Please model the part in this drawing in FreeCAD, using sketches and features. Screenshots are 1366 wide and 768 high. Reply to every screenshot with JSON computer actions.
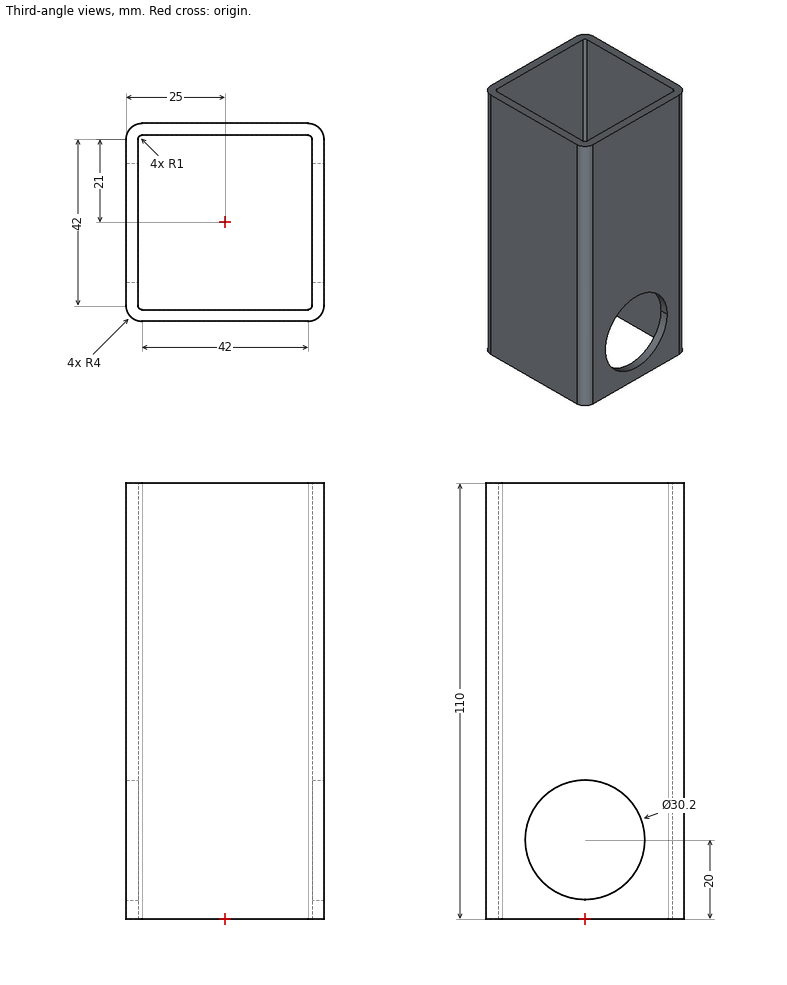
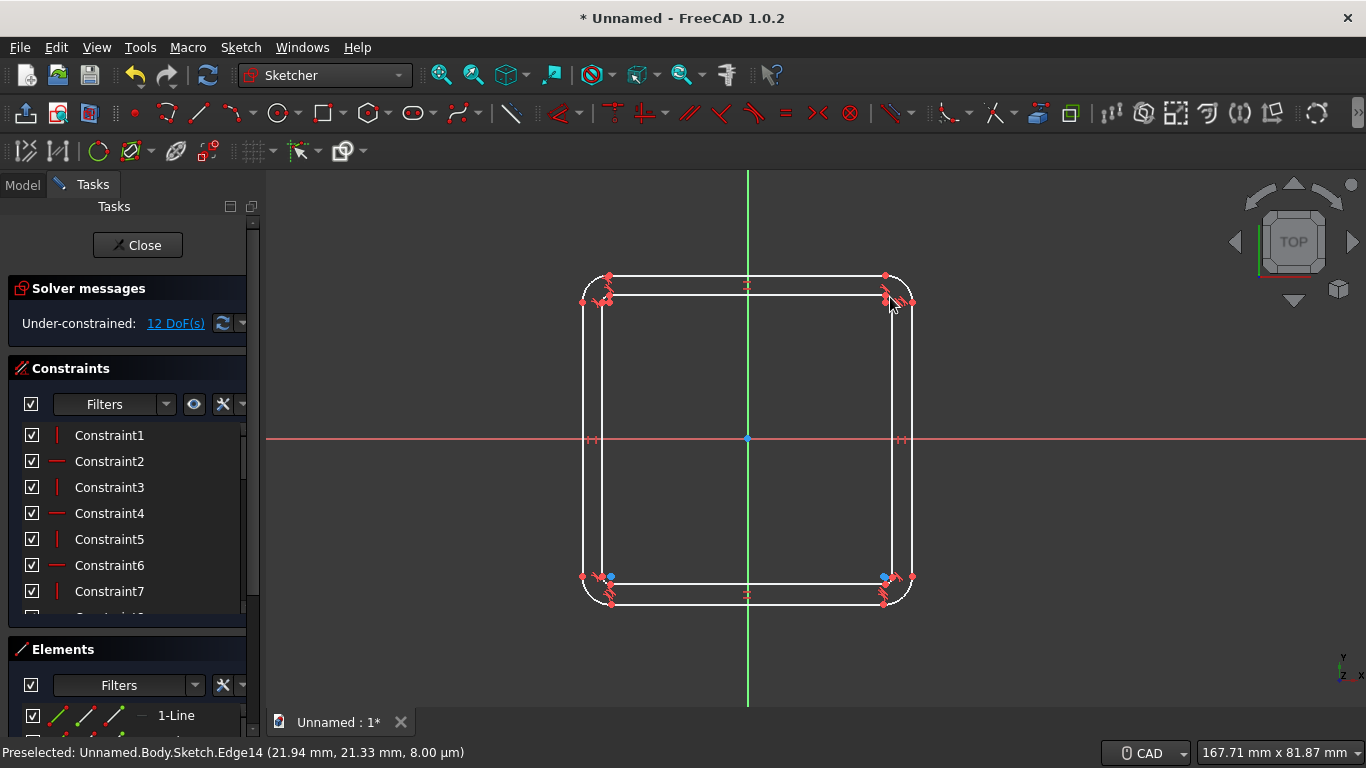
{"action": "left_click", "coordinate": [896, 602]}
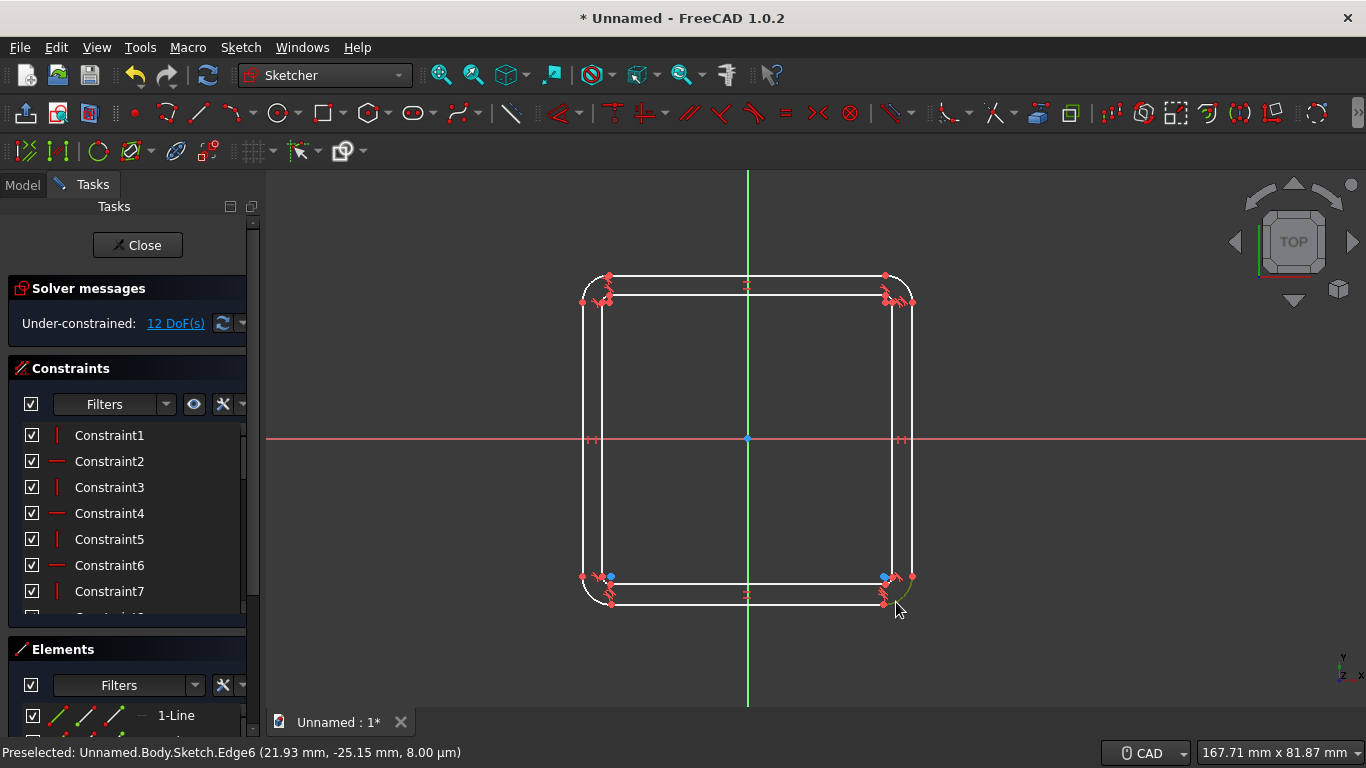
{"action": "scroll", "coordinate": [890, 582], "scroll_direction": "up", "scroll_amount": 5}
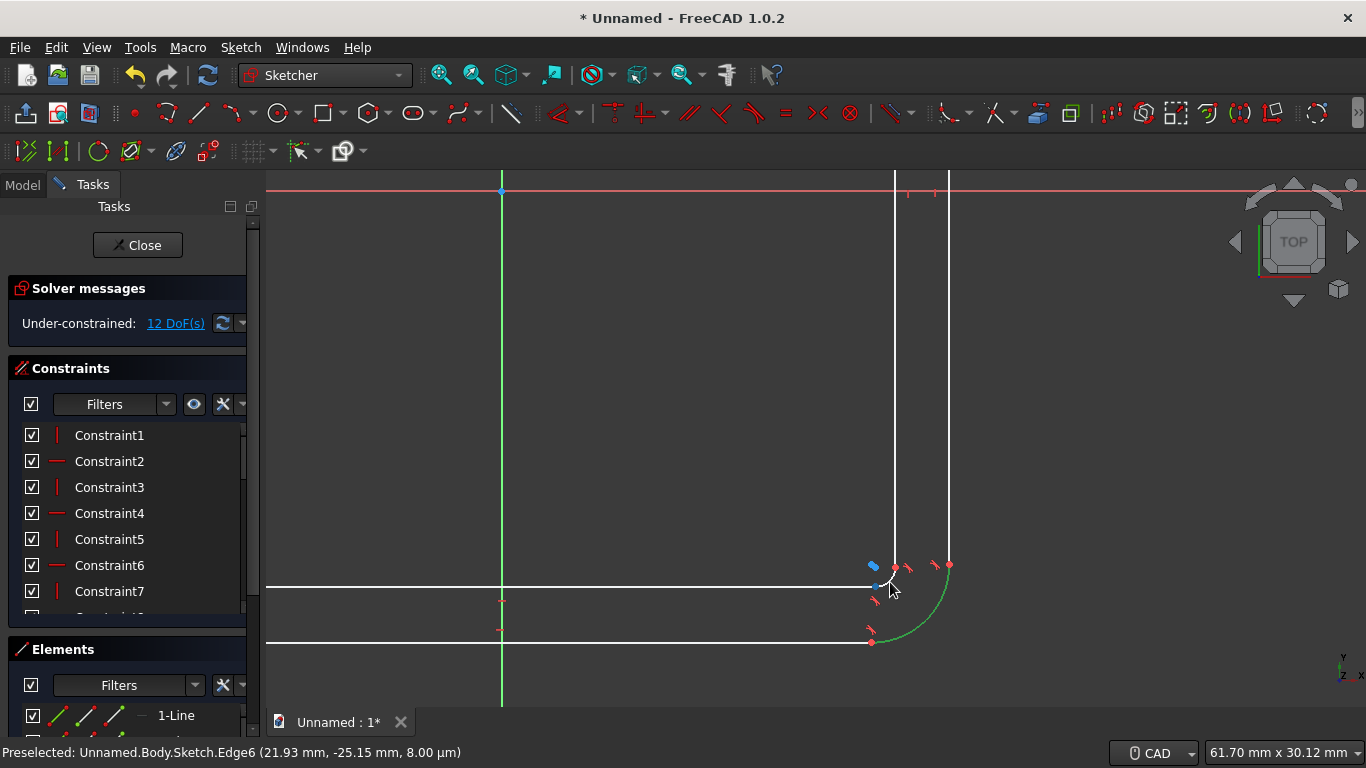
{"action": "left_click", "coordinate": [890, 581]}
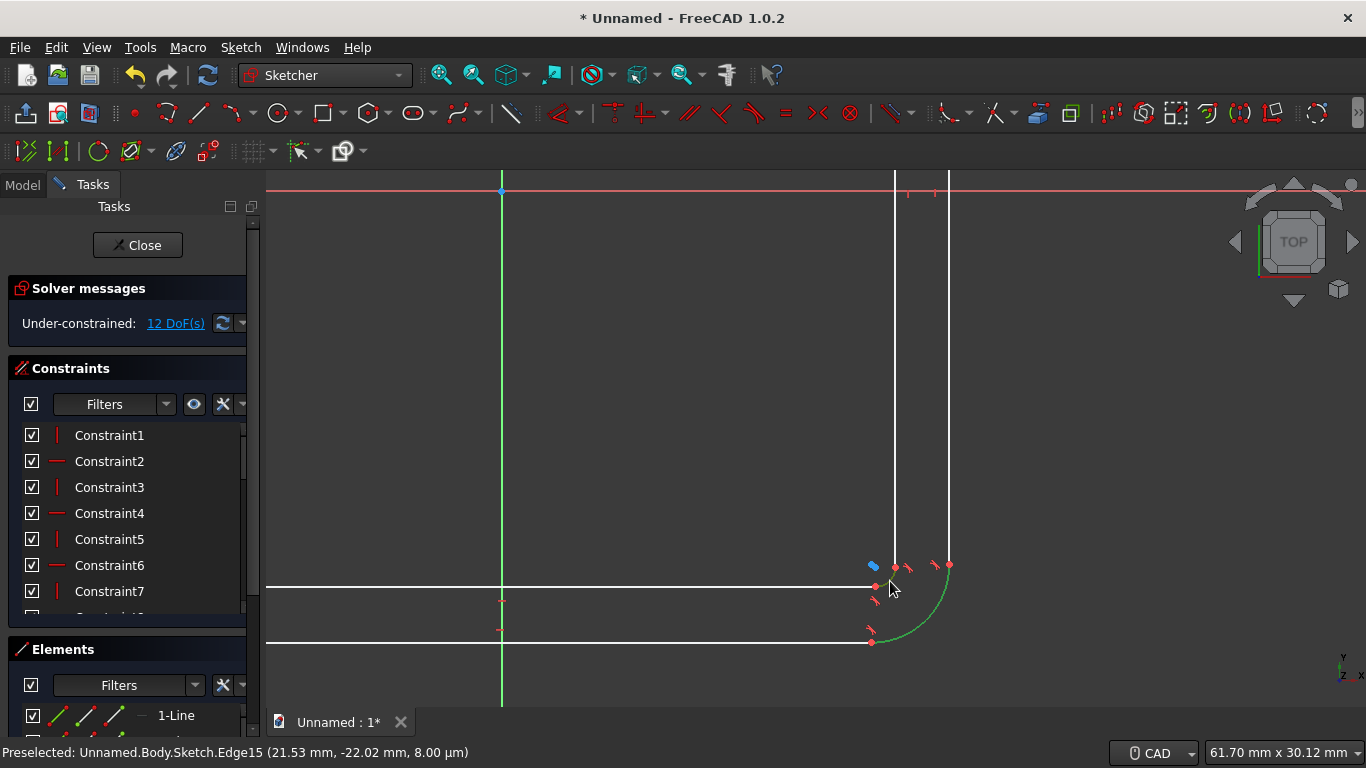
{"action": "left_click", "coordinate": [614, 114]}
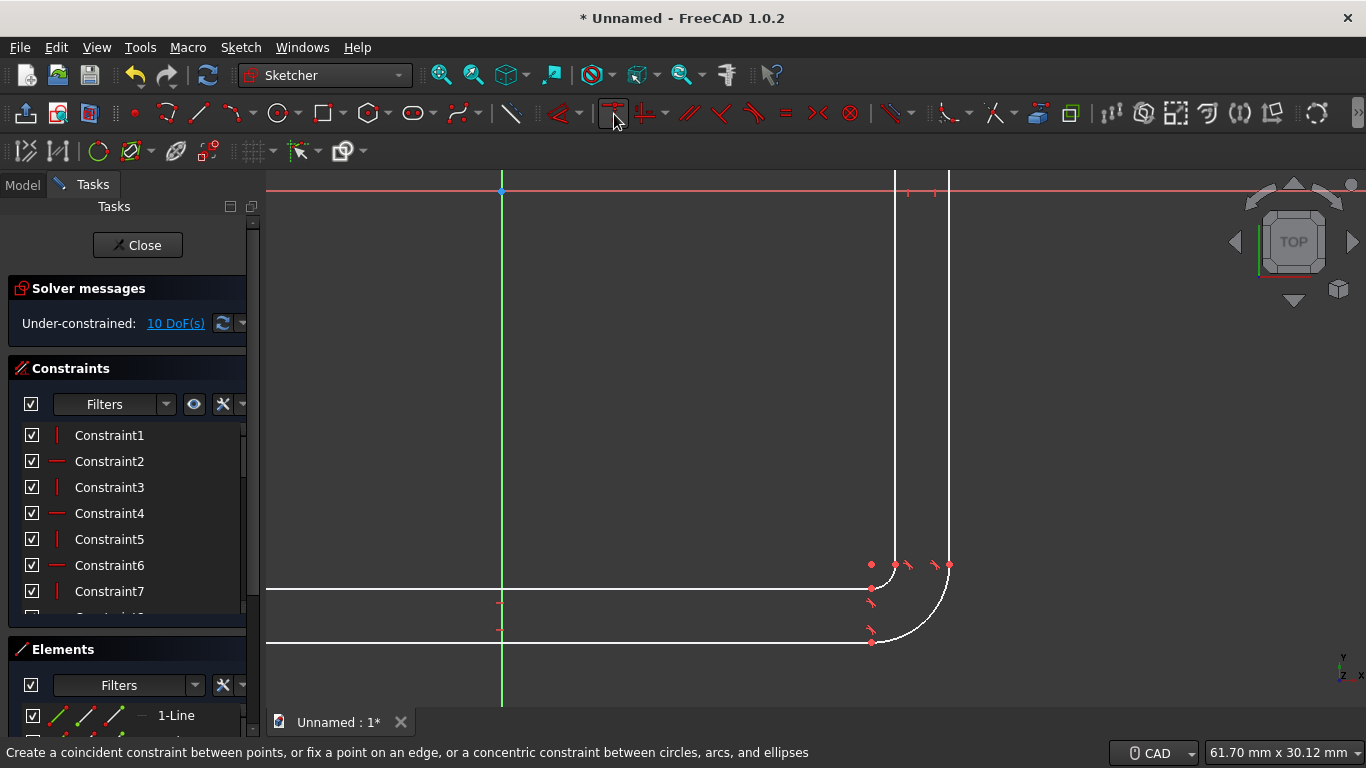
{"action": "scroll", "coordinate": [890, 582], "scroll_direction": "down", "scroll_amount": 5}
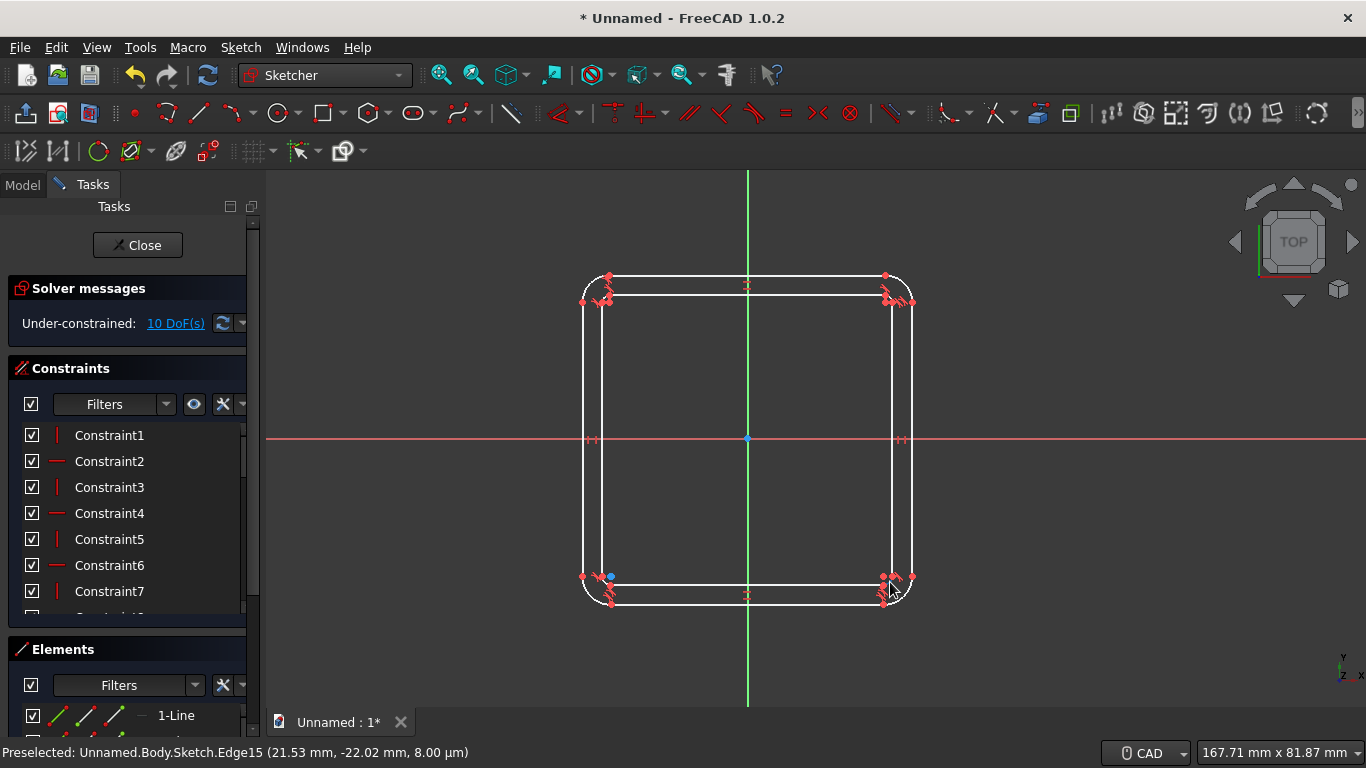
{"action": "left_click", "coordinate": [586, 589]}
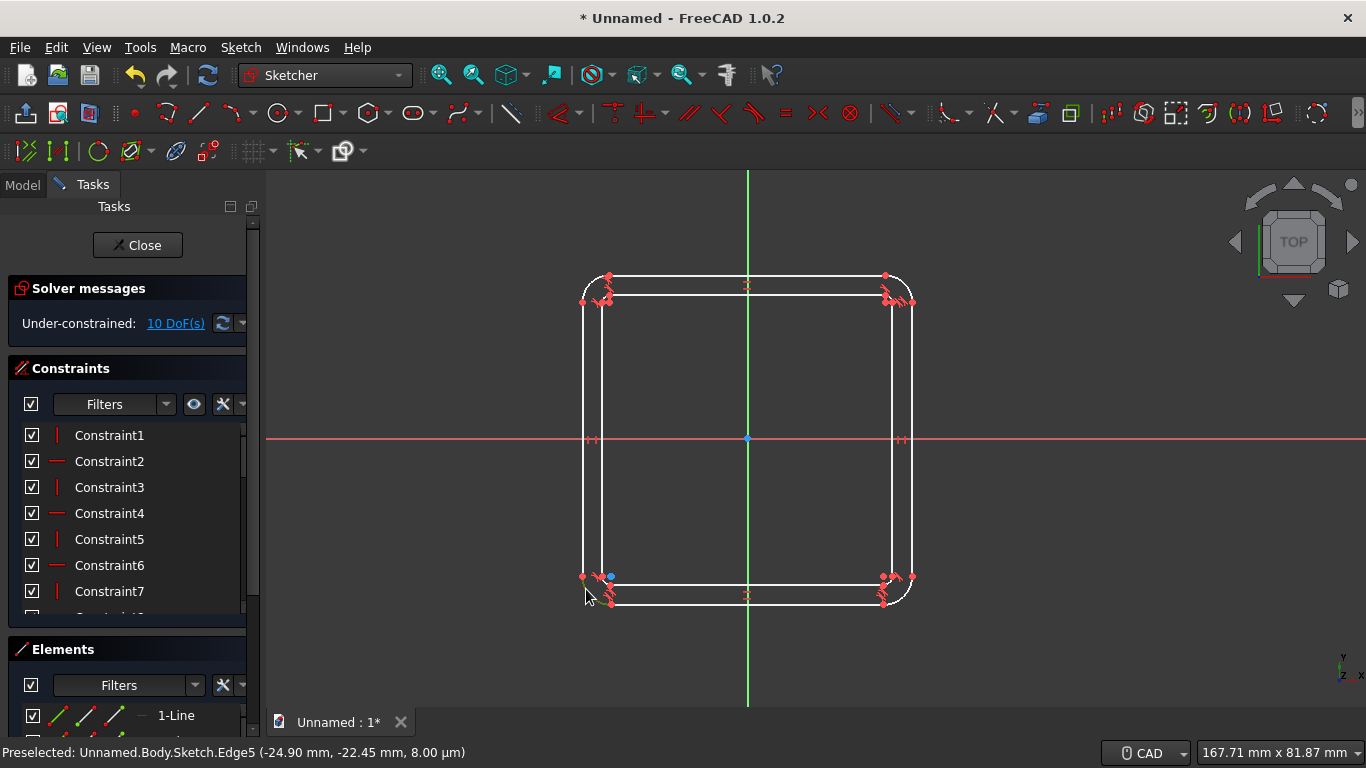
{"action": "left_click", "coordinate": [896, 602]}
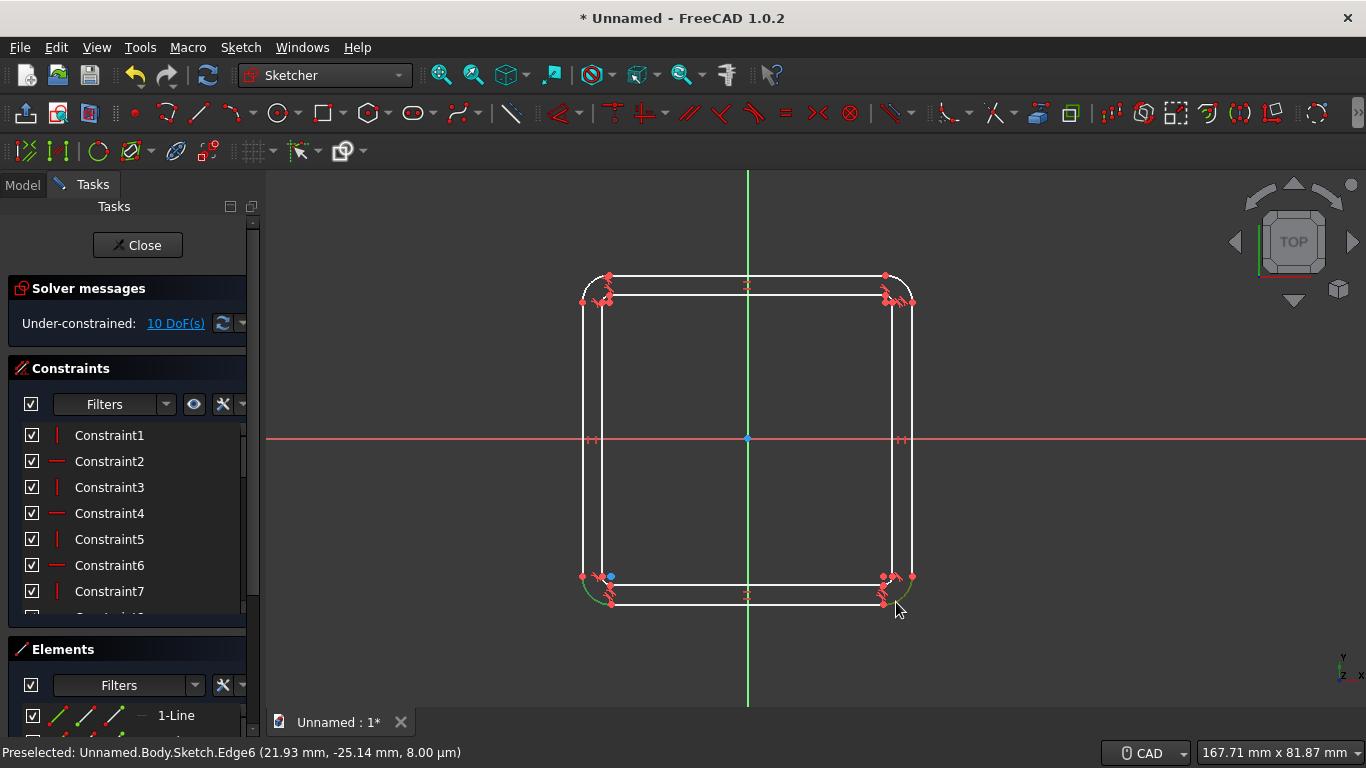
{"action": "left_click", "coordinate": [909, 290]}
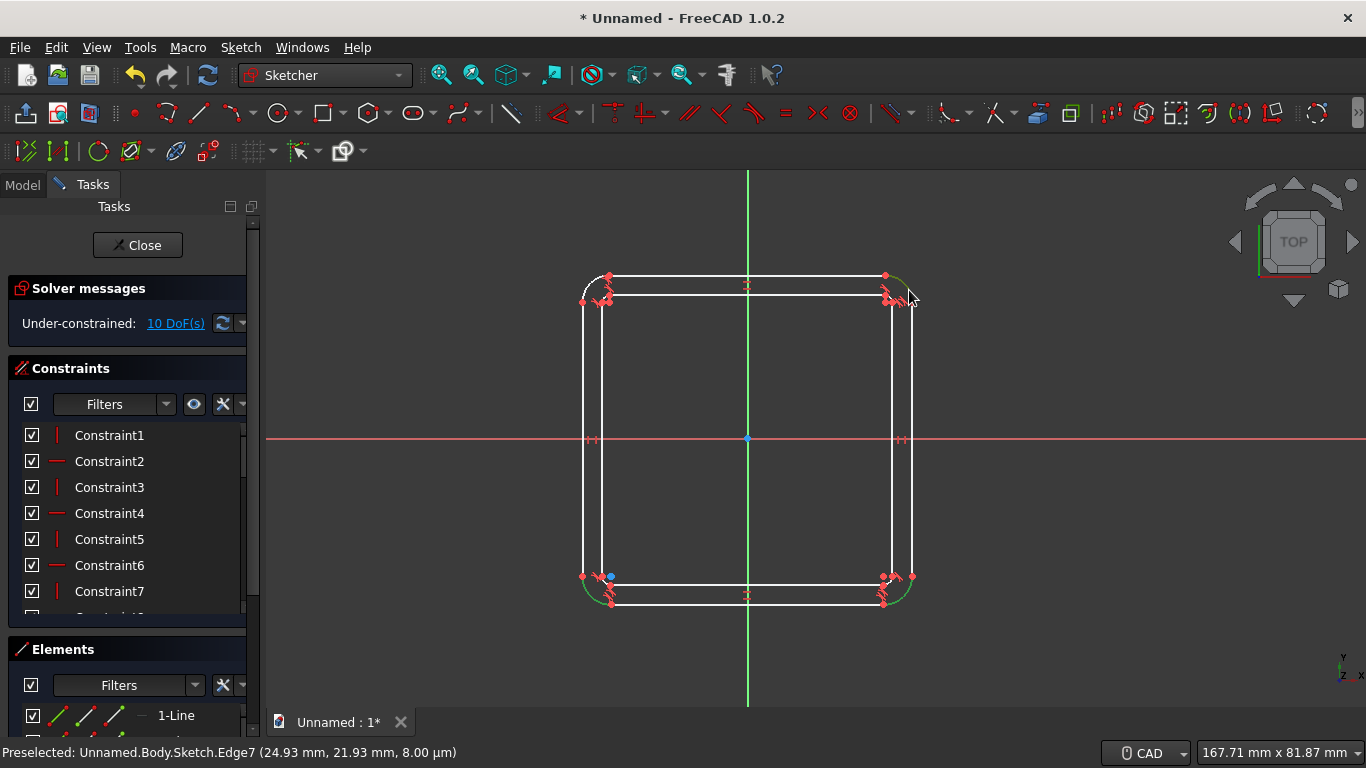
{"action": "left_click", "coordinate": [597, 278]}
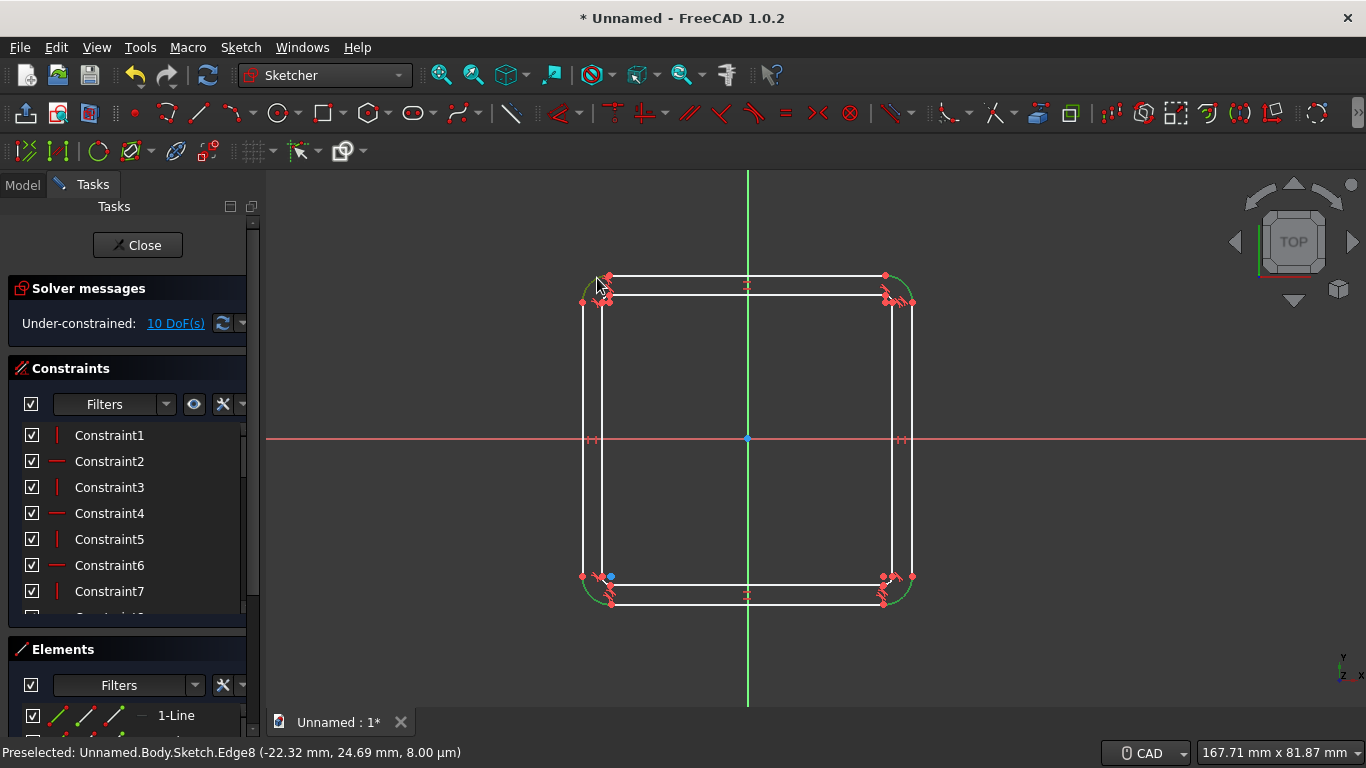
{"action": "left_click", "coordinate": [786, 114]}